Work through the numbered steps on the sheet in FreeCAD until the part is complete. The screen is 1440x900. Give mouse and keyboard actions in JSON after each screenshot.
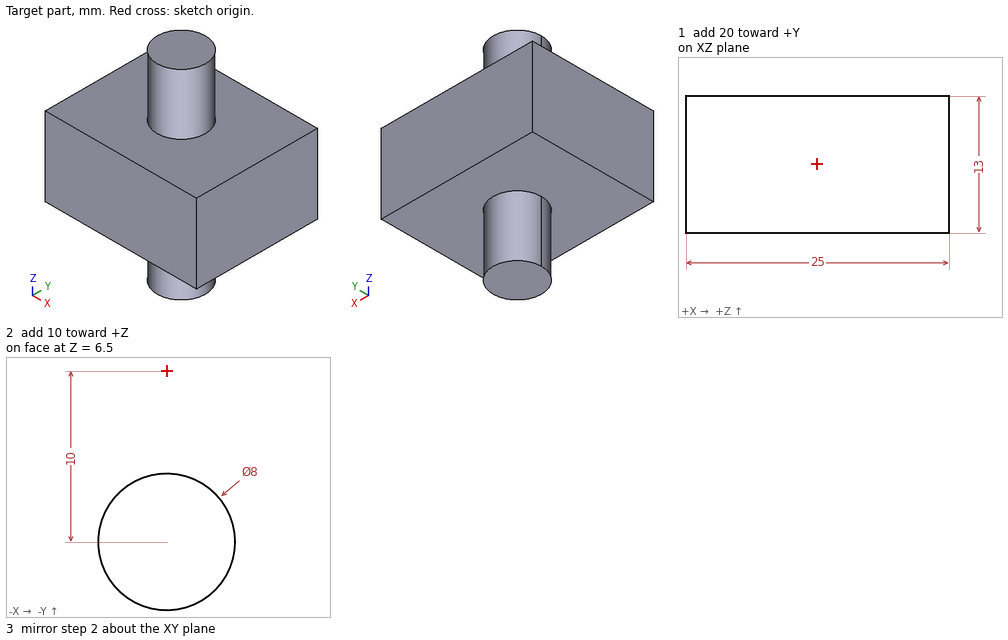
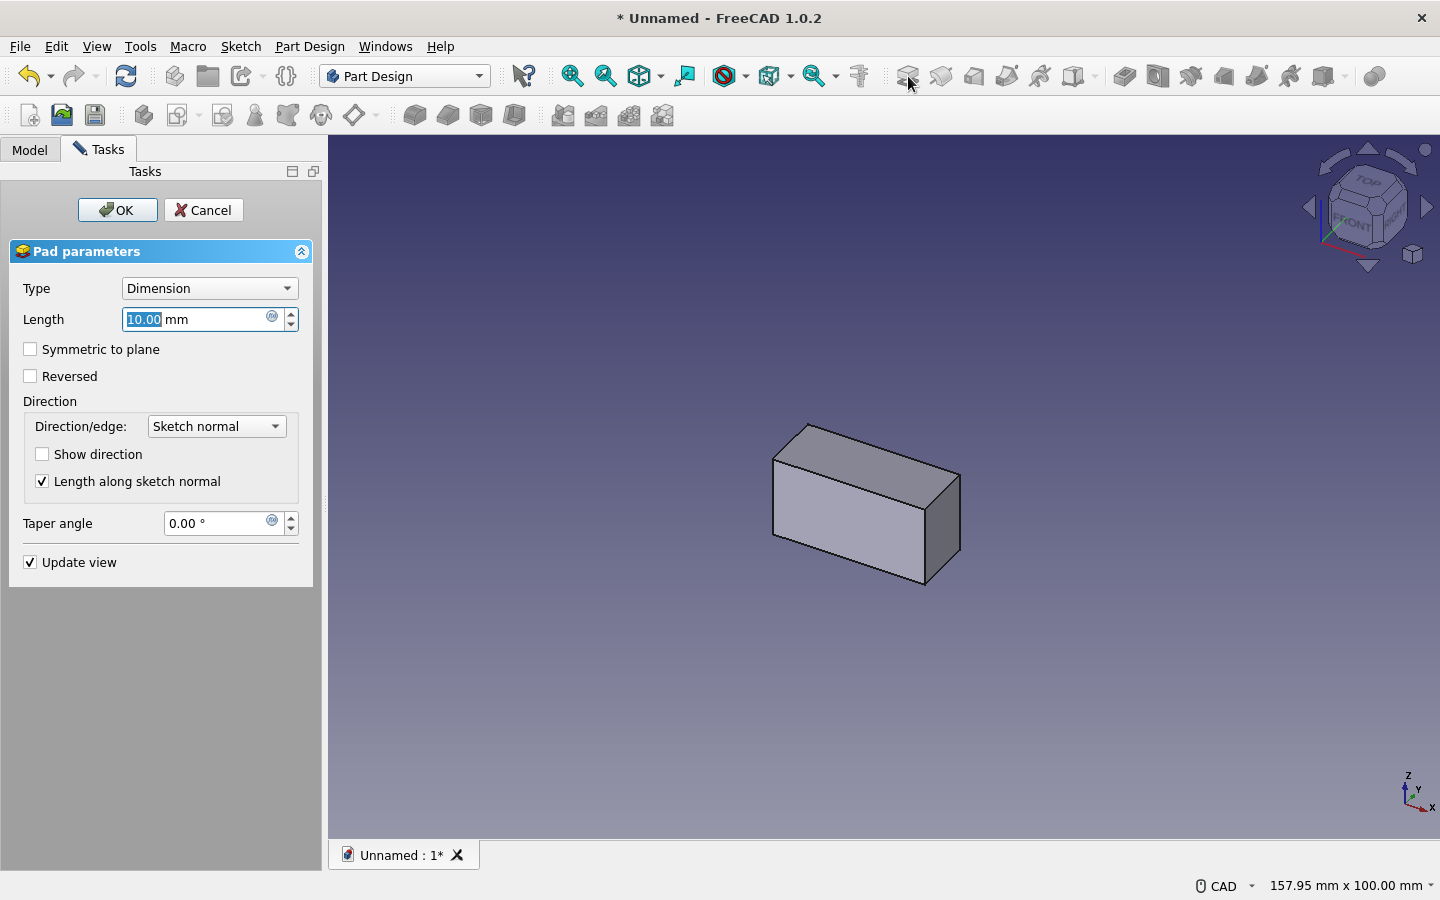
{"action": "type", "text": "20"}
{"action": "key", "text": "Tab"}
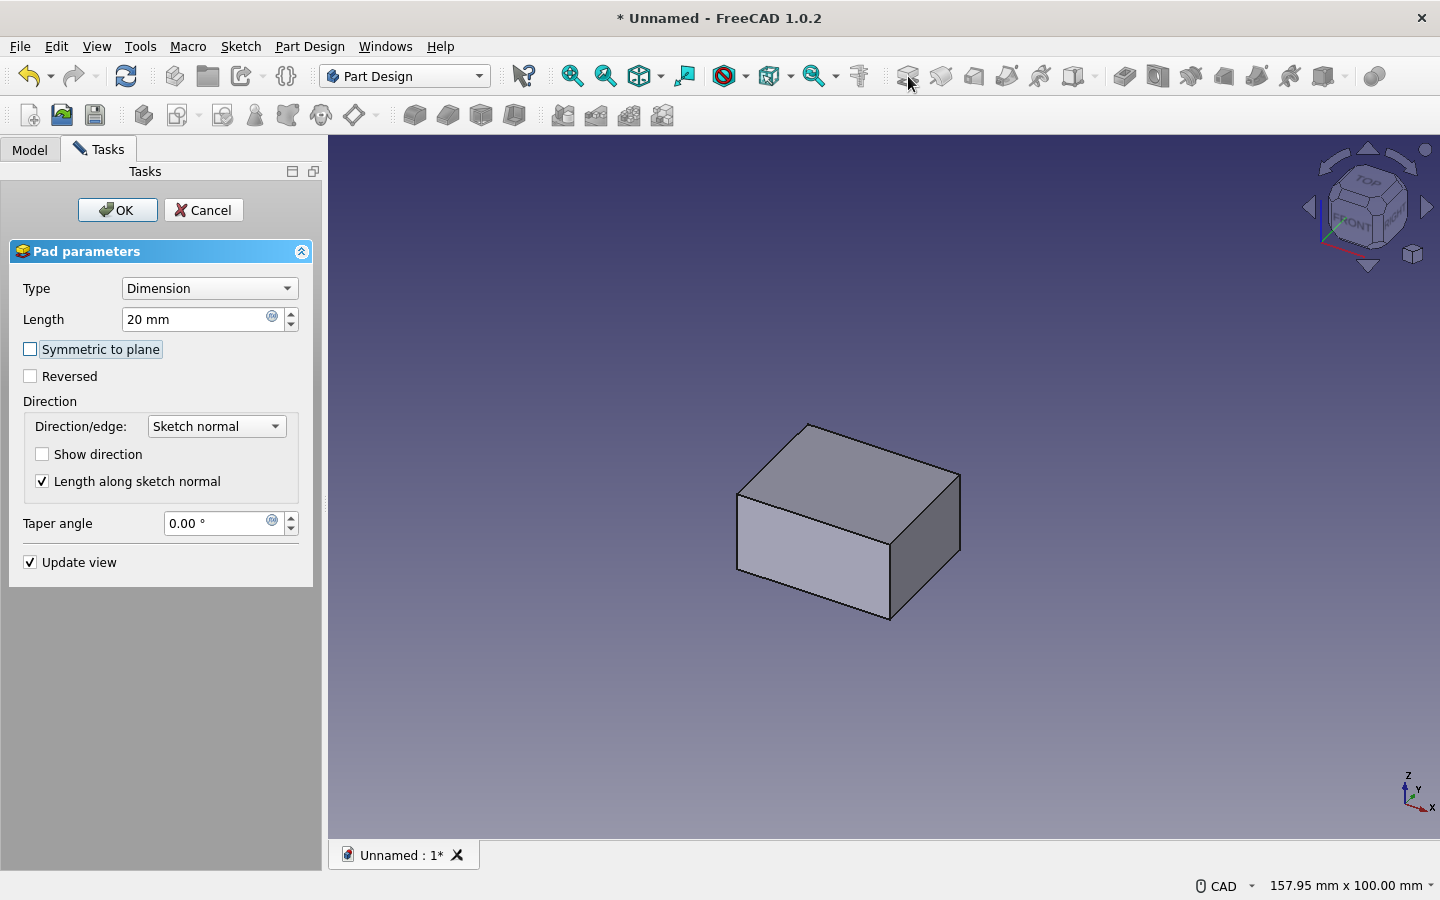
{"action": "left_click", "coordinate": [31, 376]}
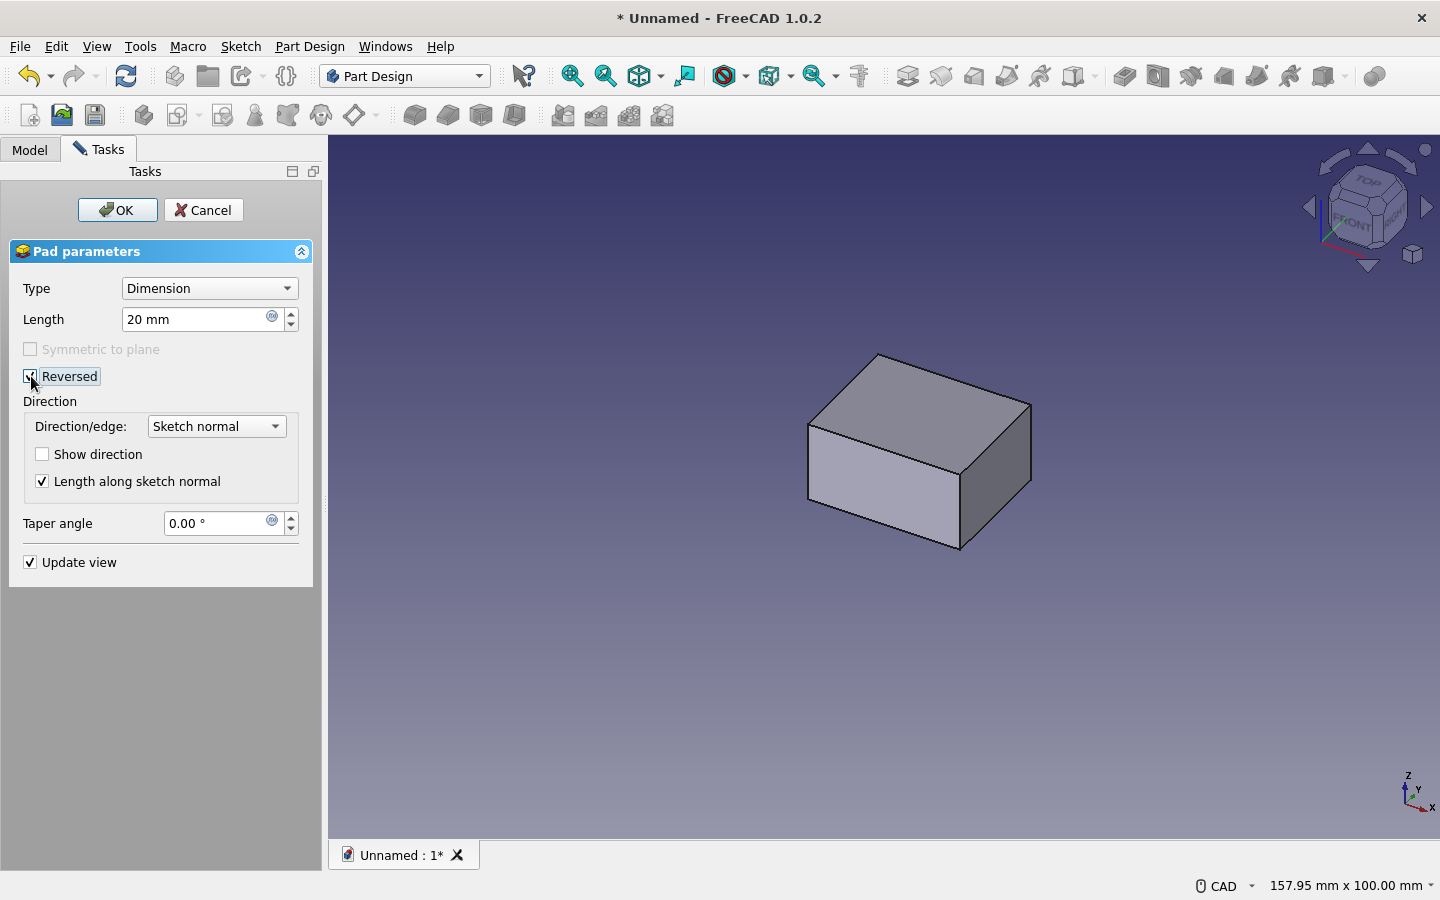
{"action": "left_click", "coordinate": [118, 210]}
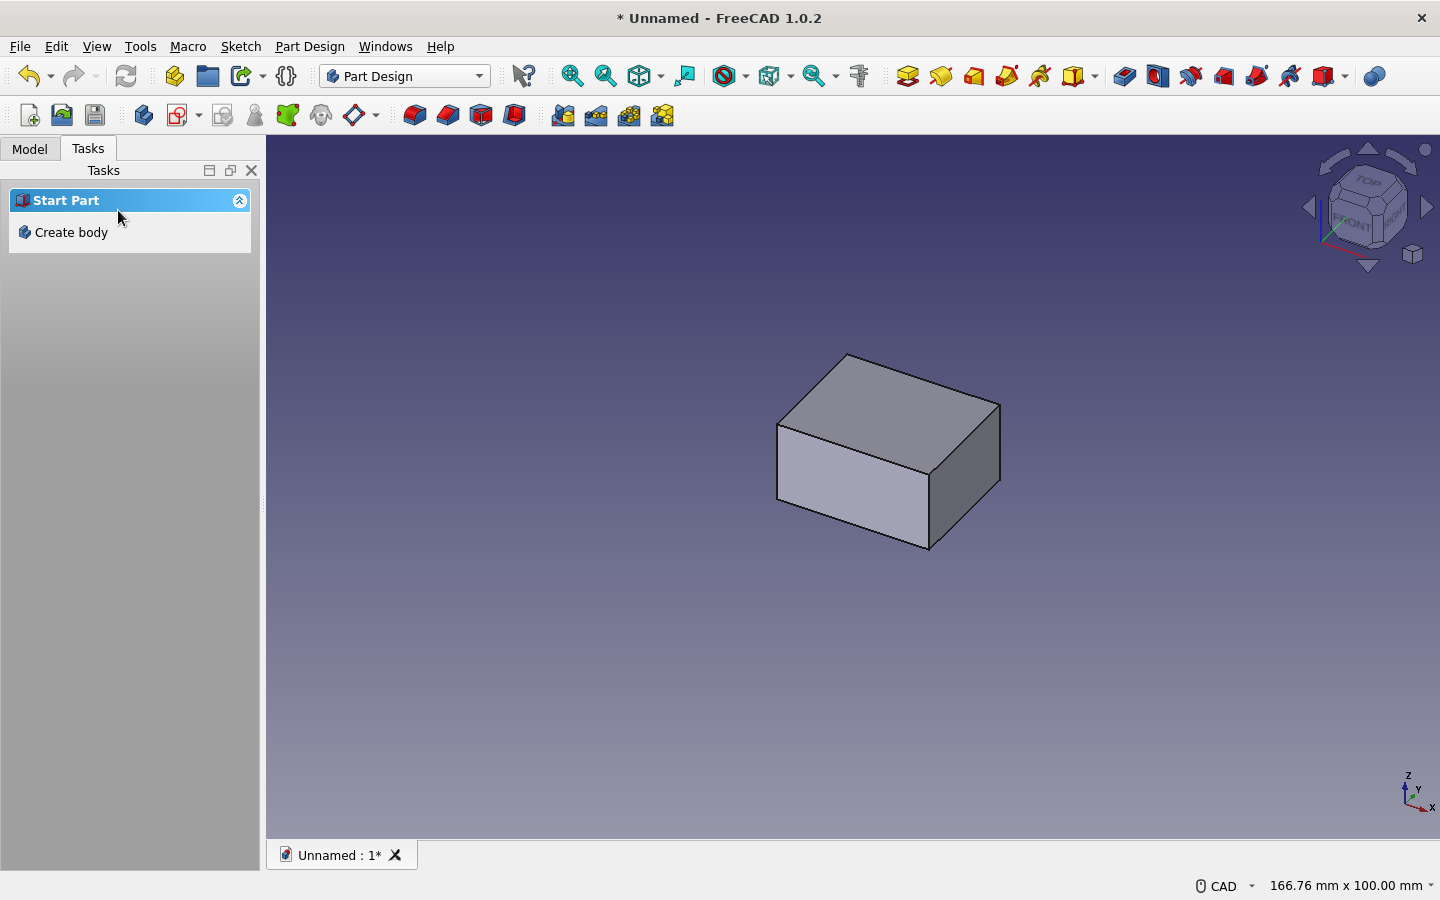
{"action": "key", "text": "v f"}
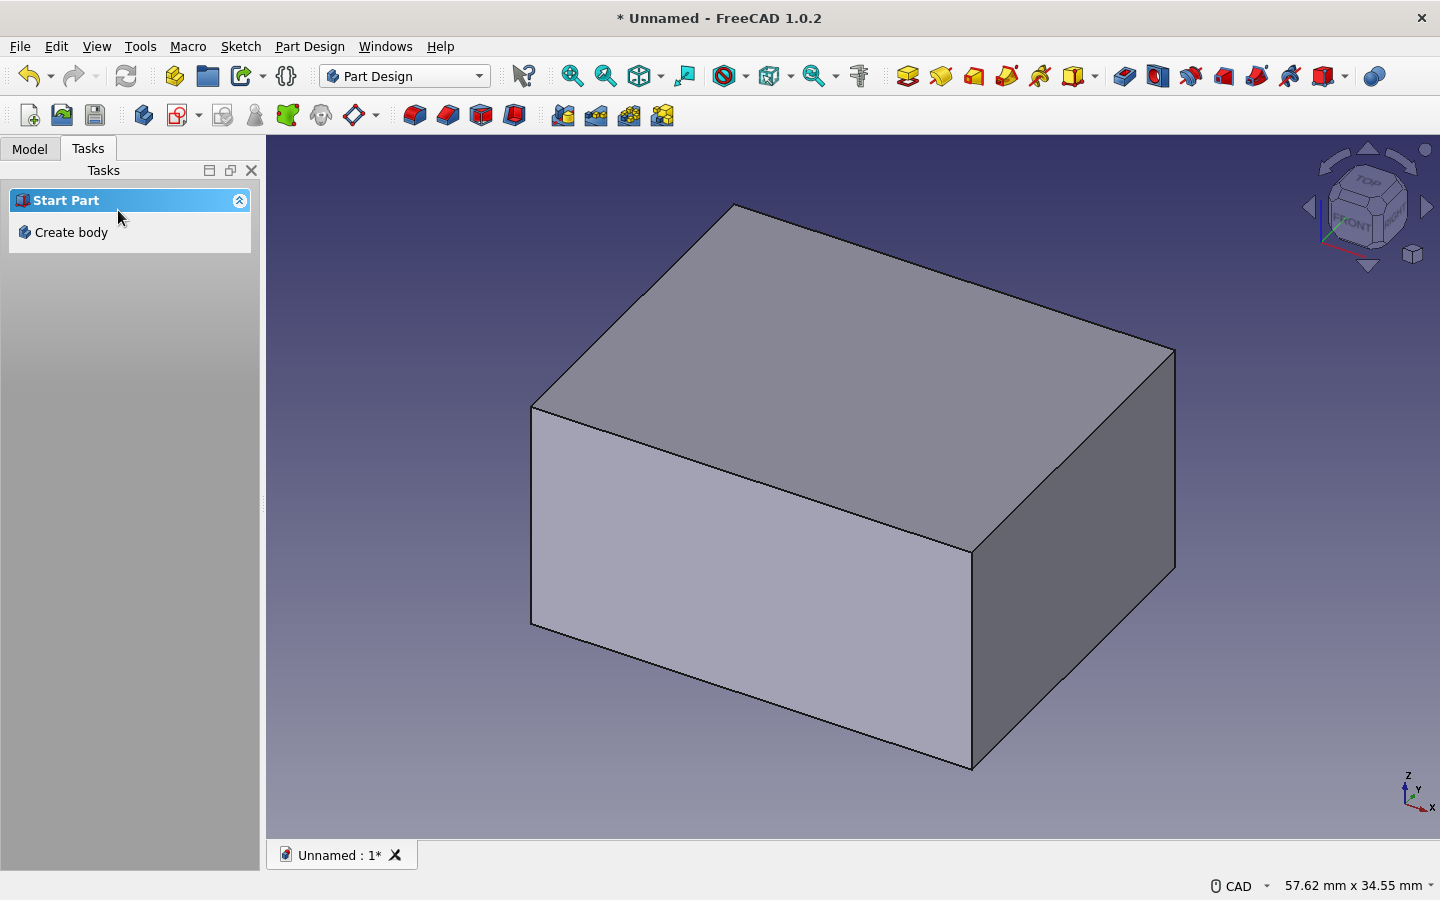
{"action": "left_click", "coordinate": [853, 378]}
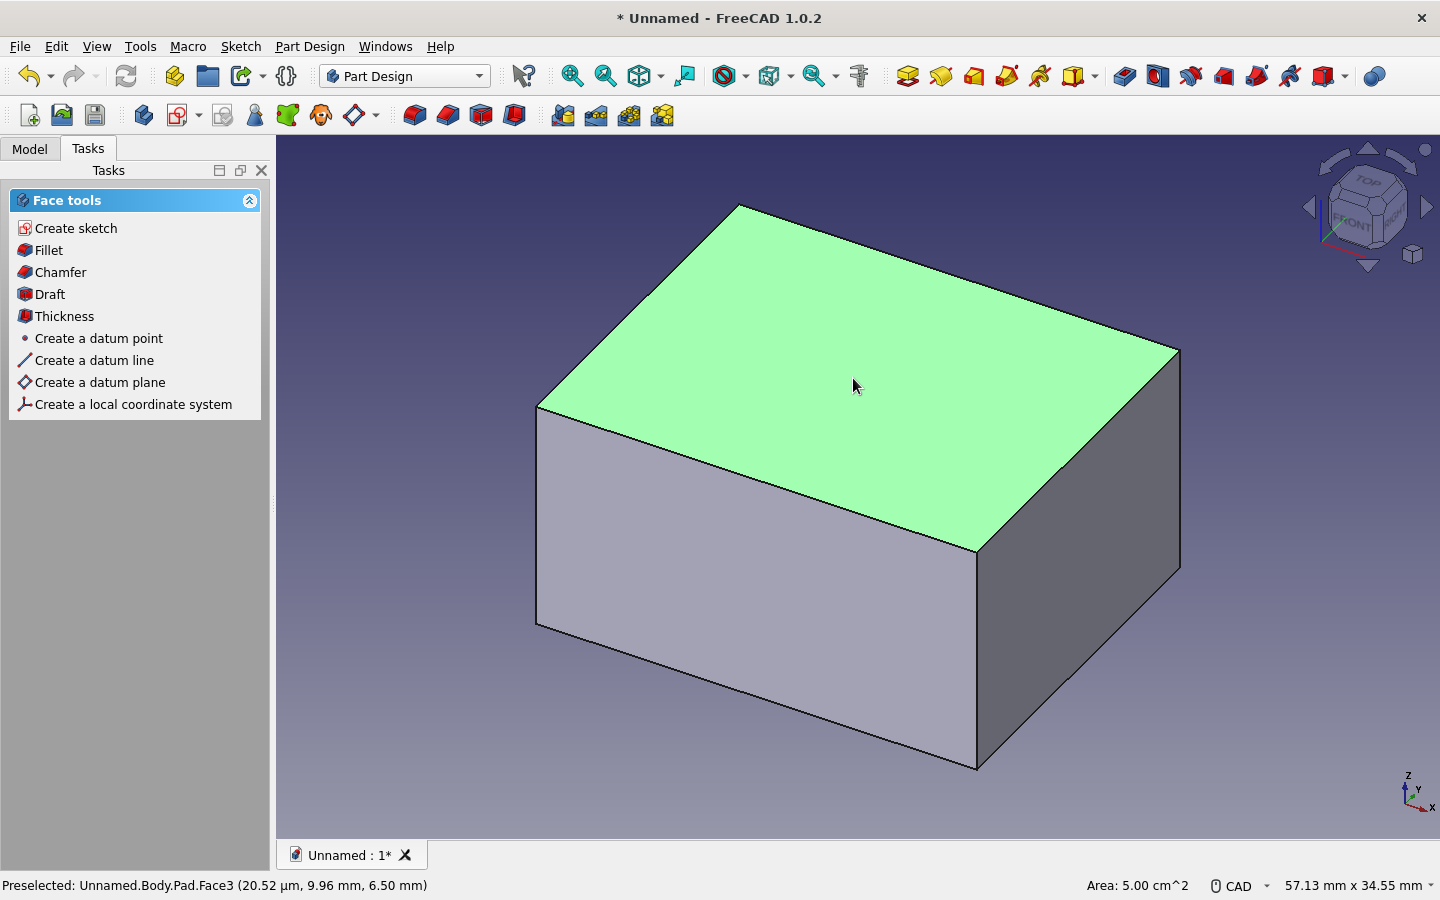
{"action": "left_click", "coordinate": [176, 116]}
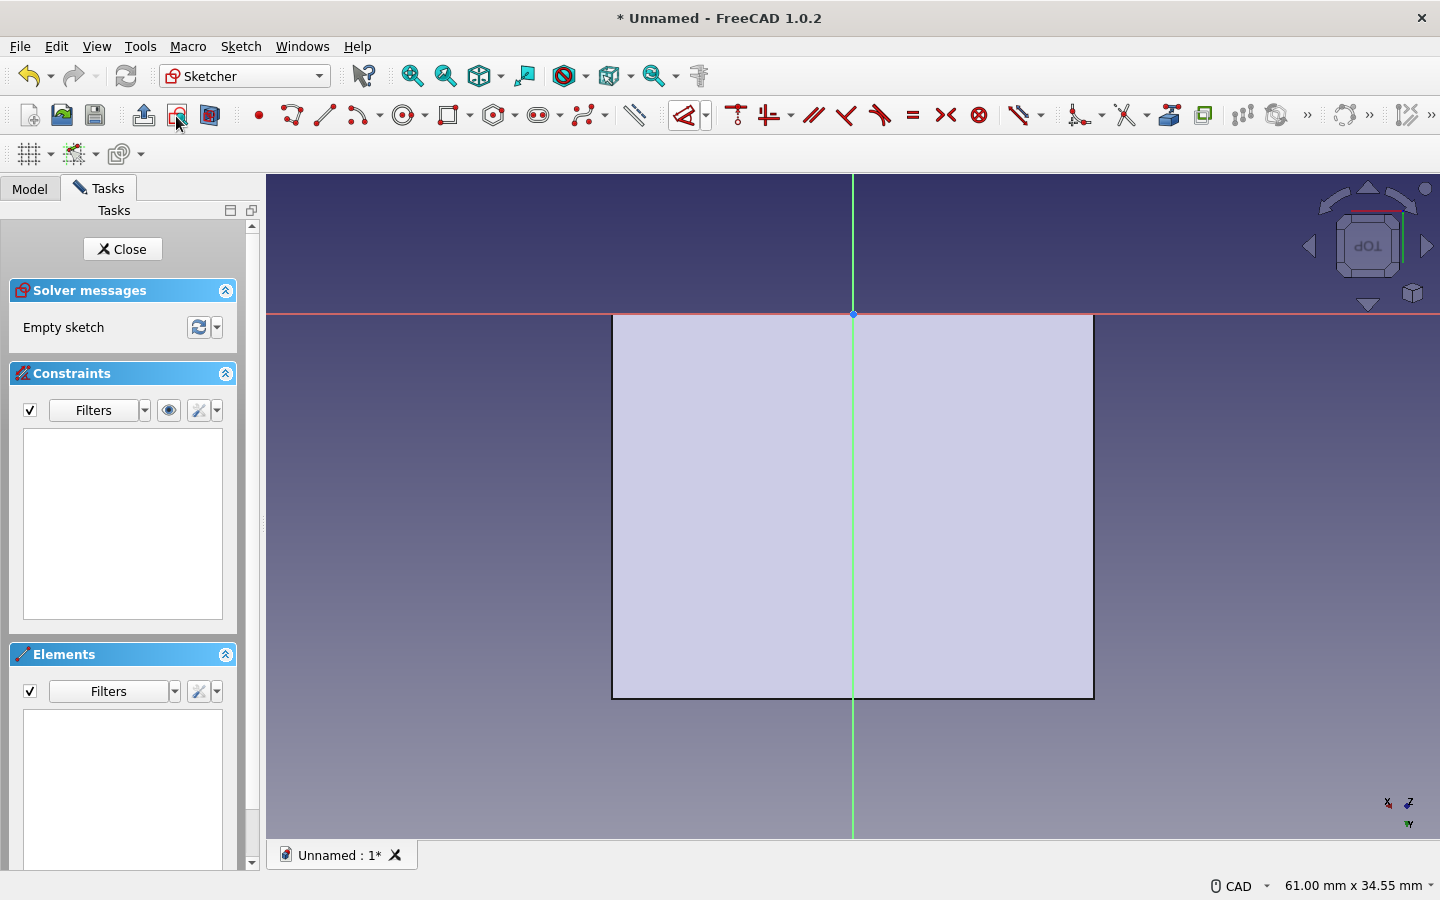
{"action": "scroll", "coordinate": [992, 331], "scroll_direction": "up", "scroll_amount": 2}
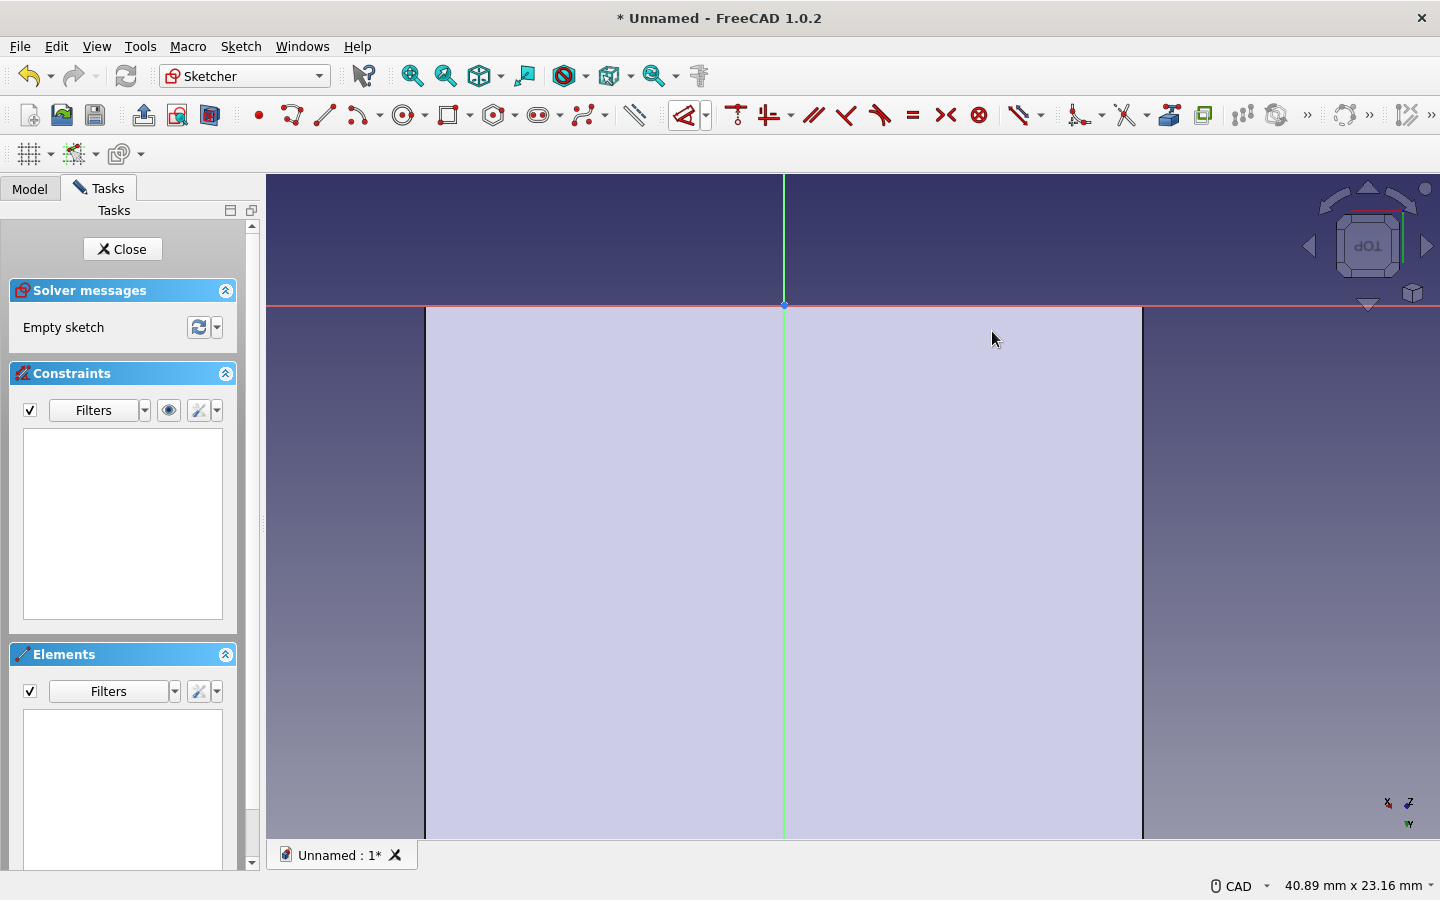
{"action": "key", "text": "g c"}